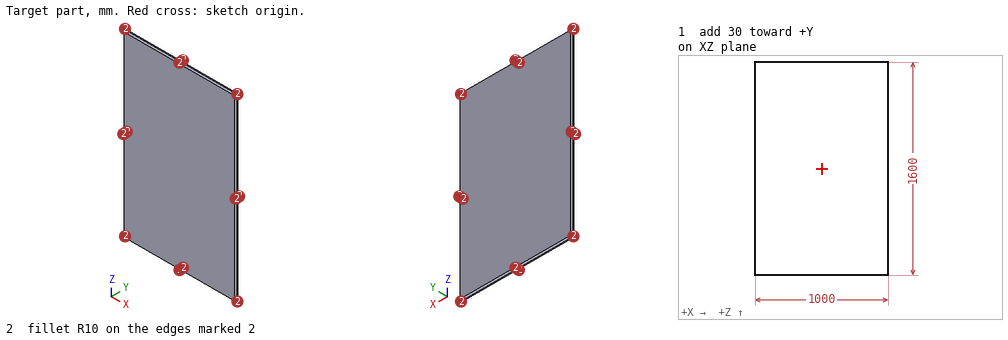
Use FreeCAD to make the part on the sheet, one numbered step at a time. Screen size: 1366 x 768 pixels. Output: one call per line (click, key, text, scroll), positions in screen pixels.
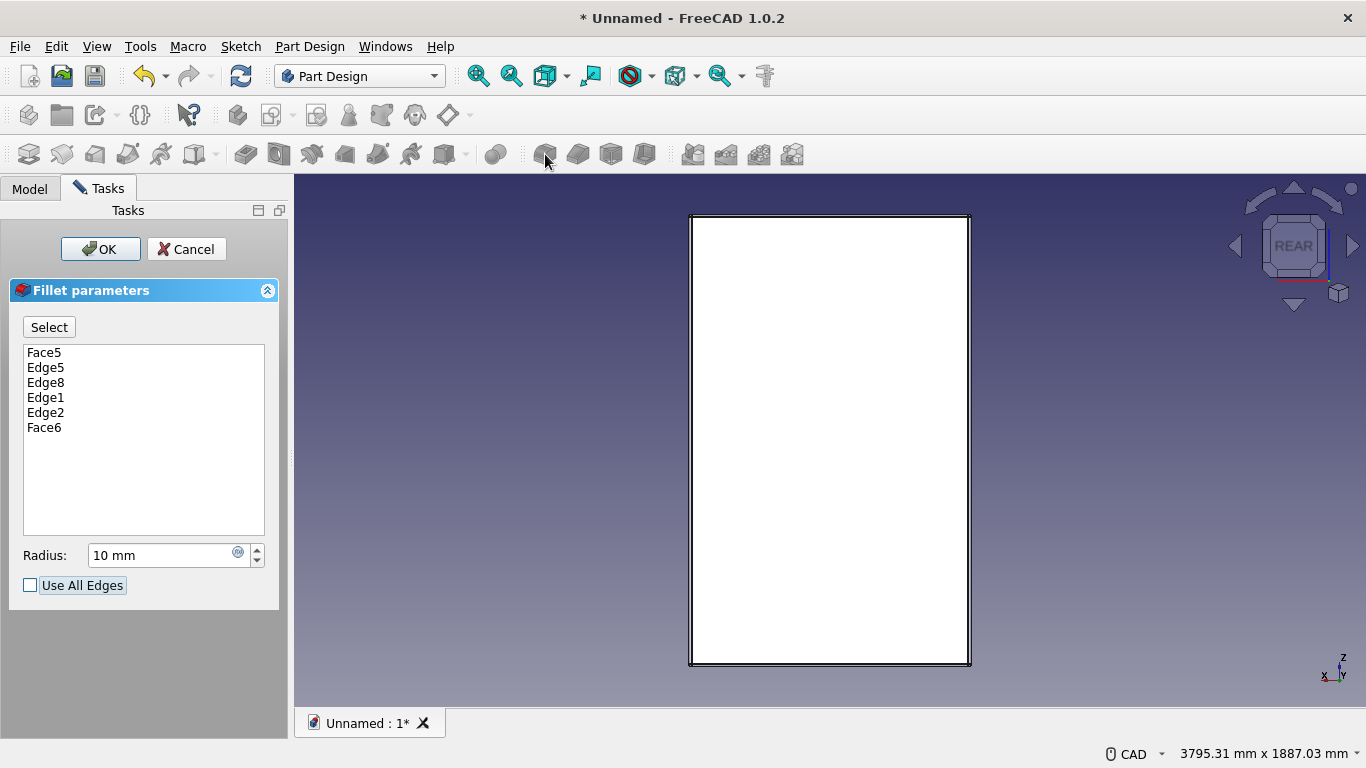
click(101, 249)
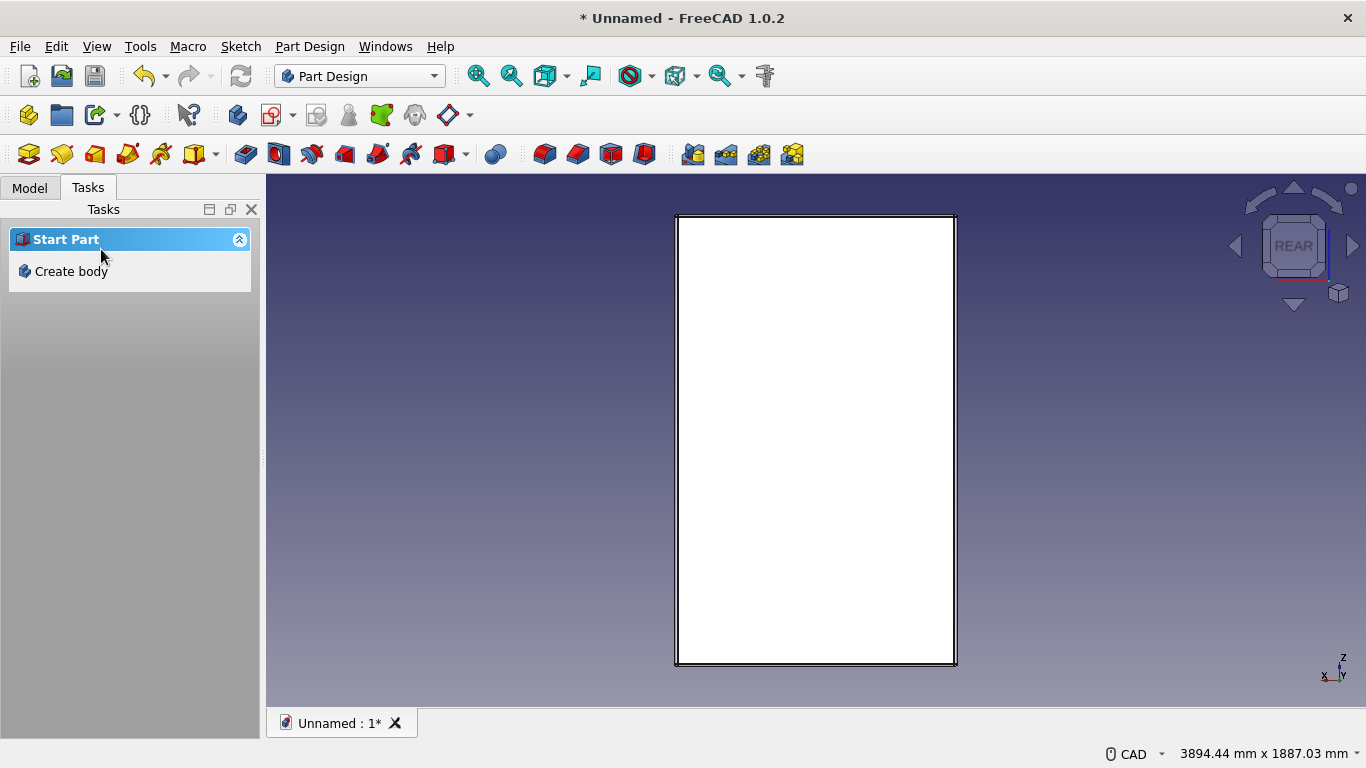
key(0)